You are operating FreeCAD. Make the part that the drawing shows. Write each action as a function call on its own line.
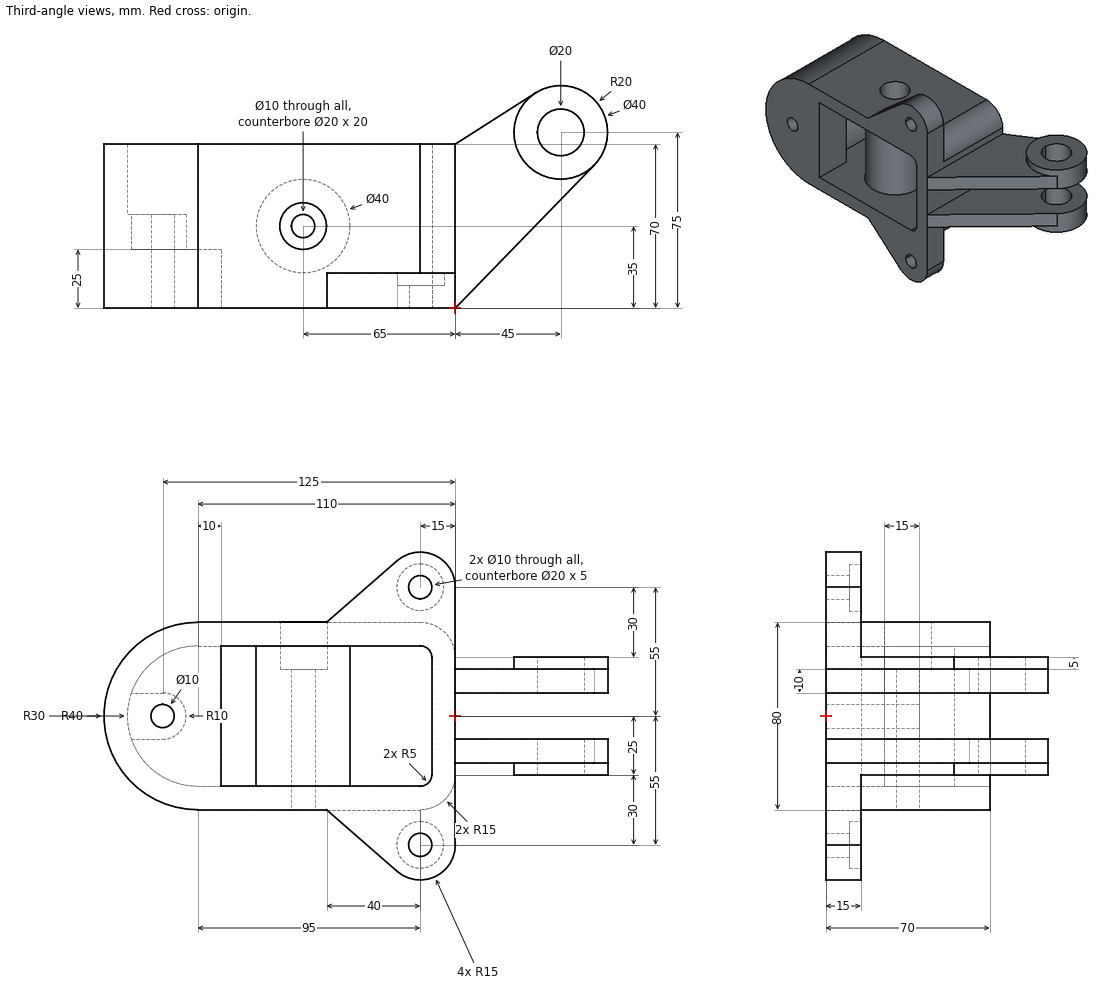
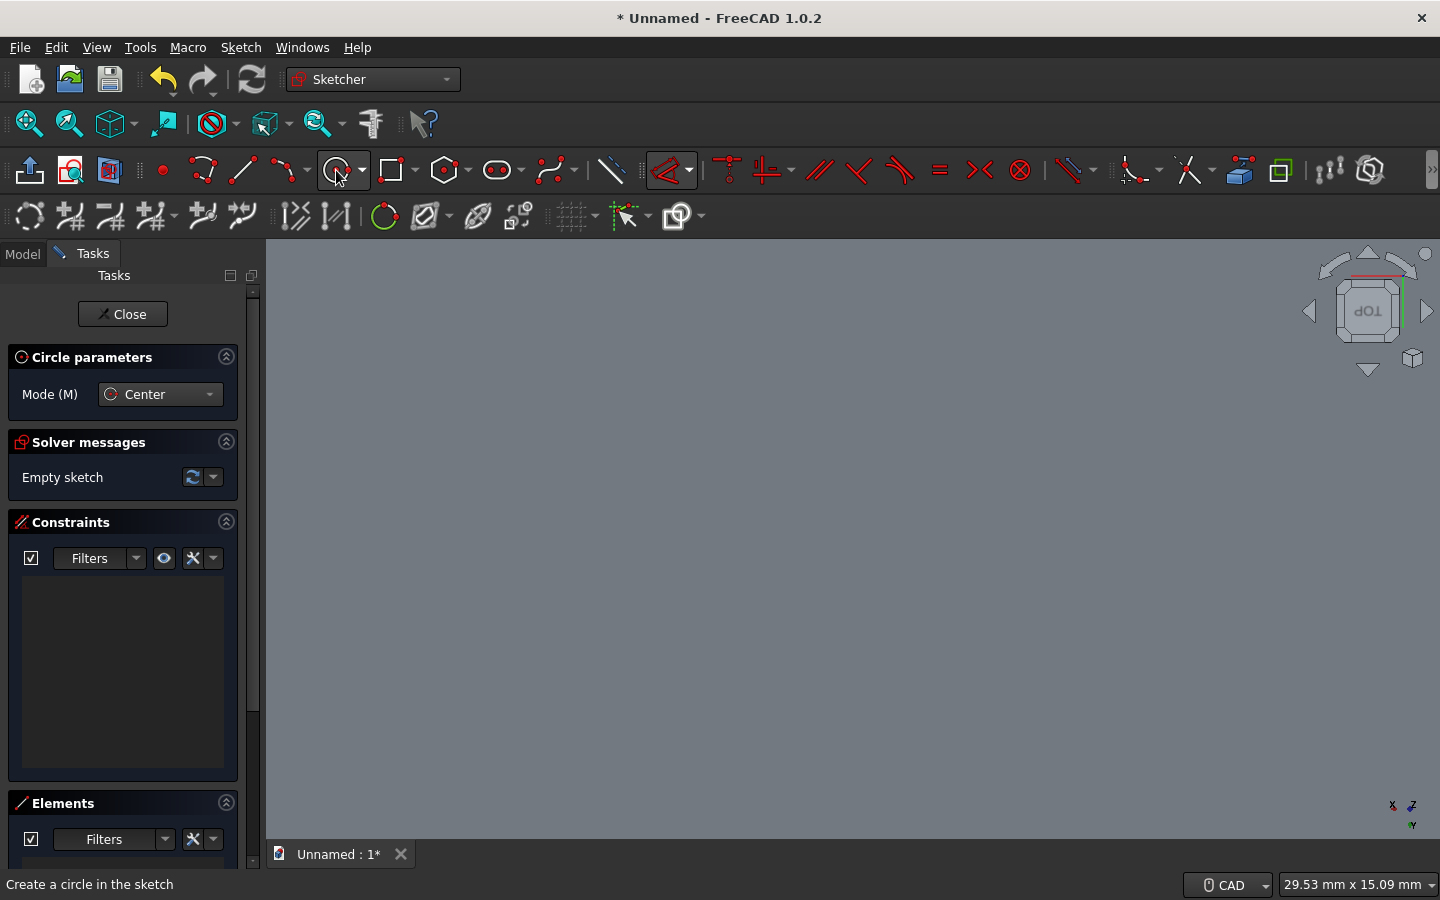
click(773, 535)
move(913, 395)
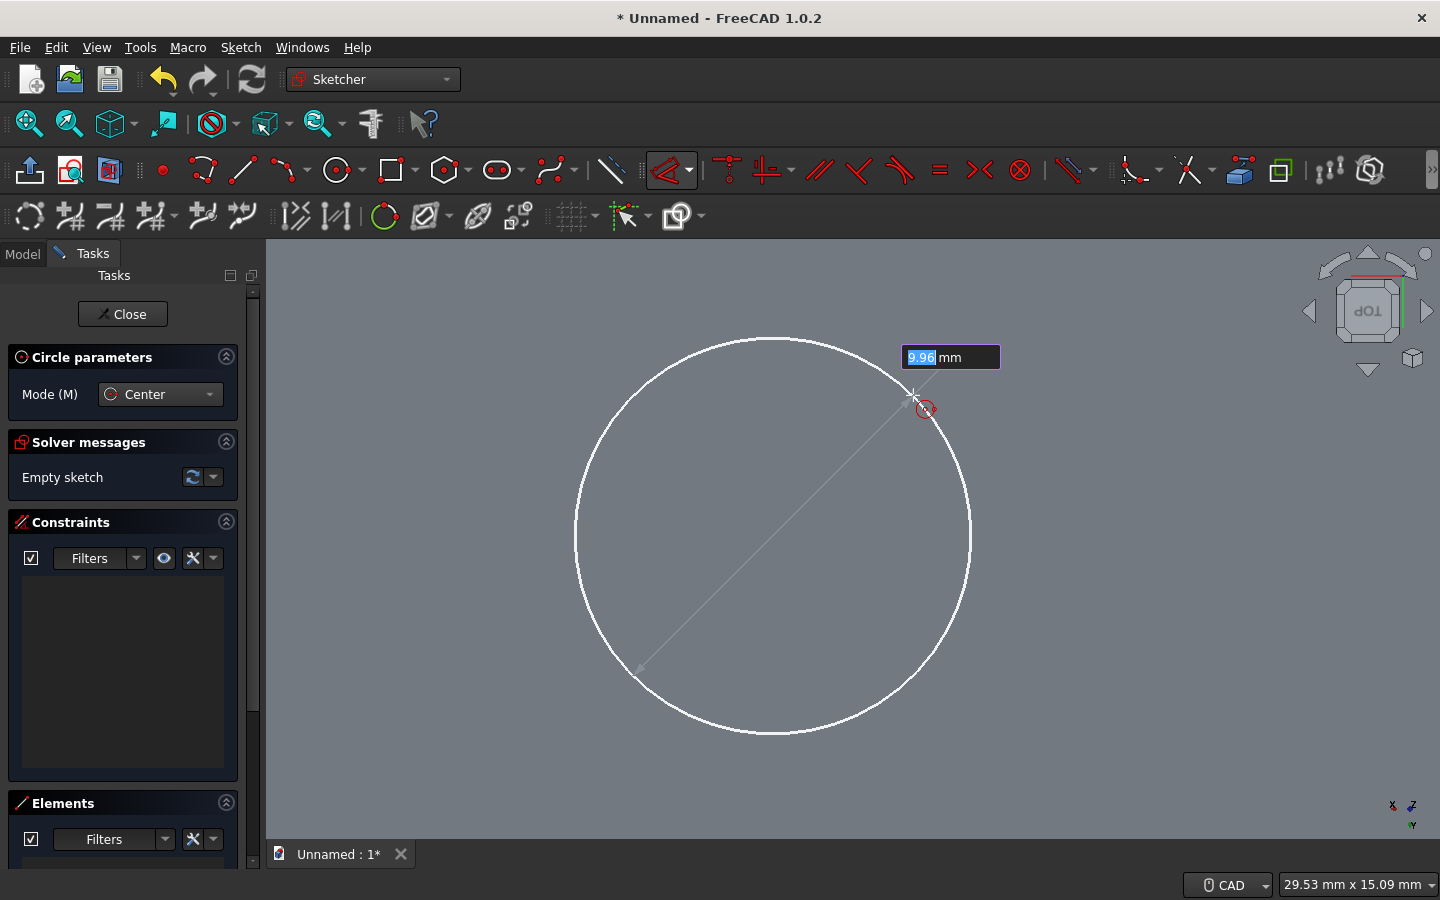
text(10)
key(Return)
key(Escape)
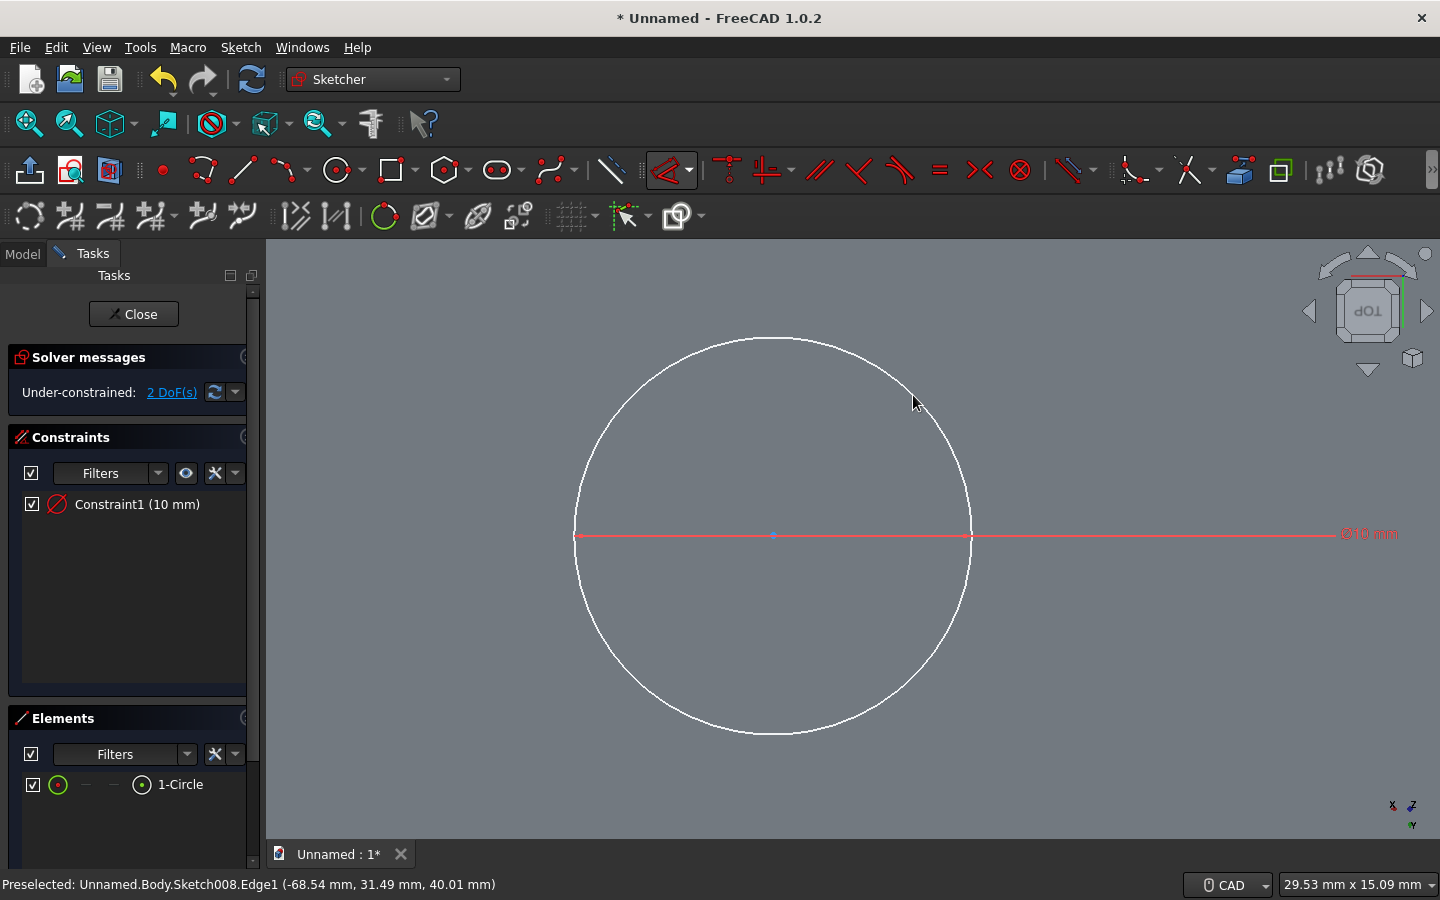
click(773, 536)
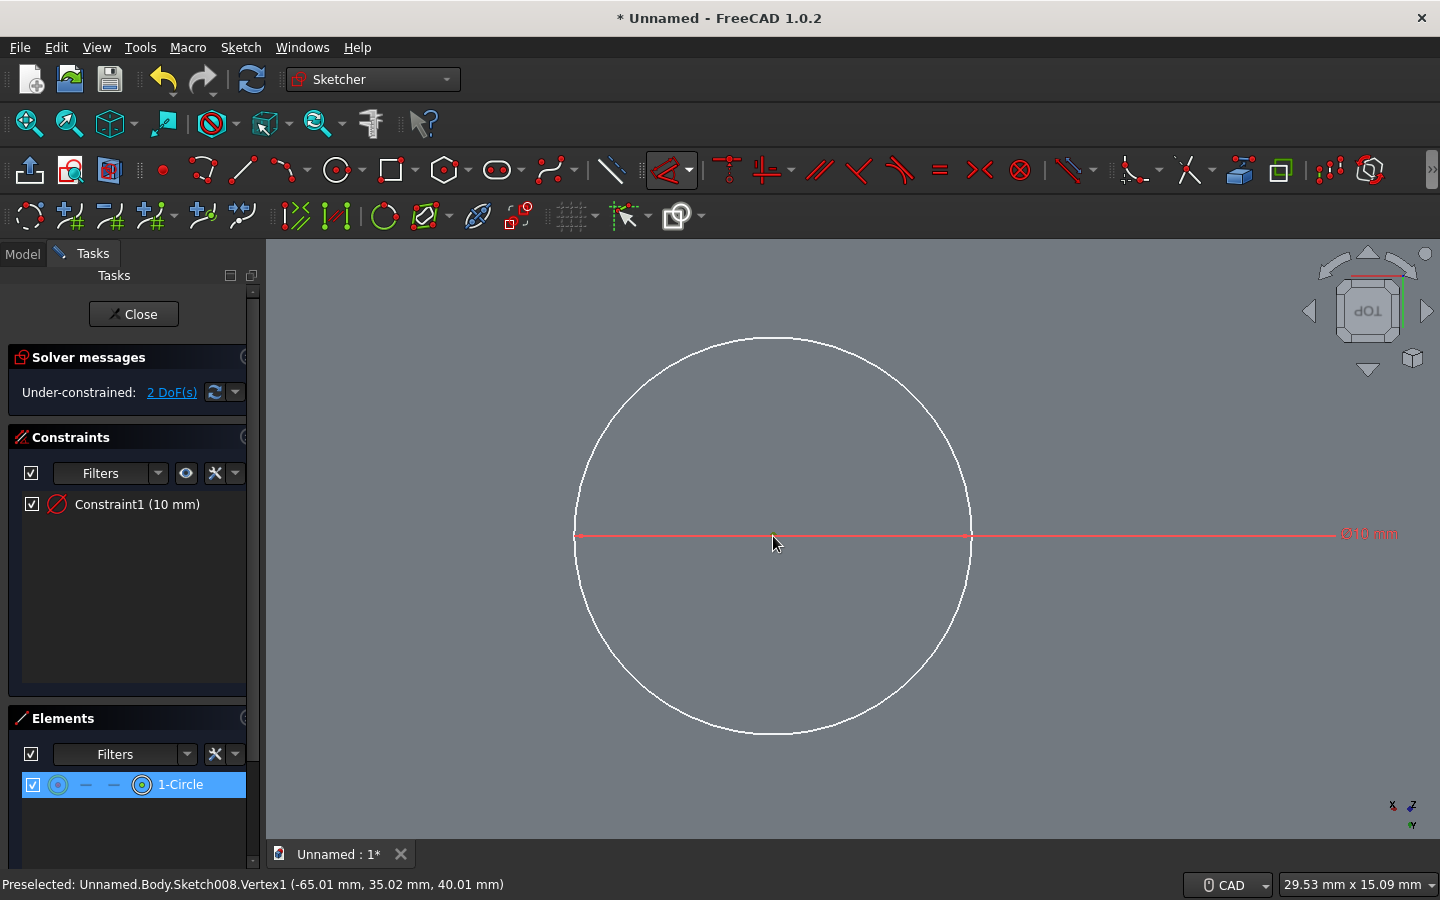
key(l)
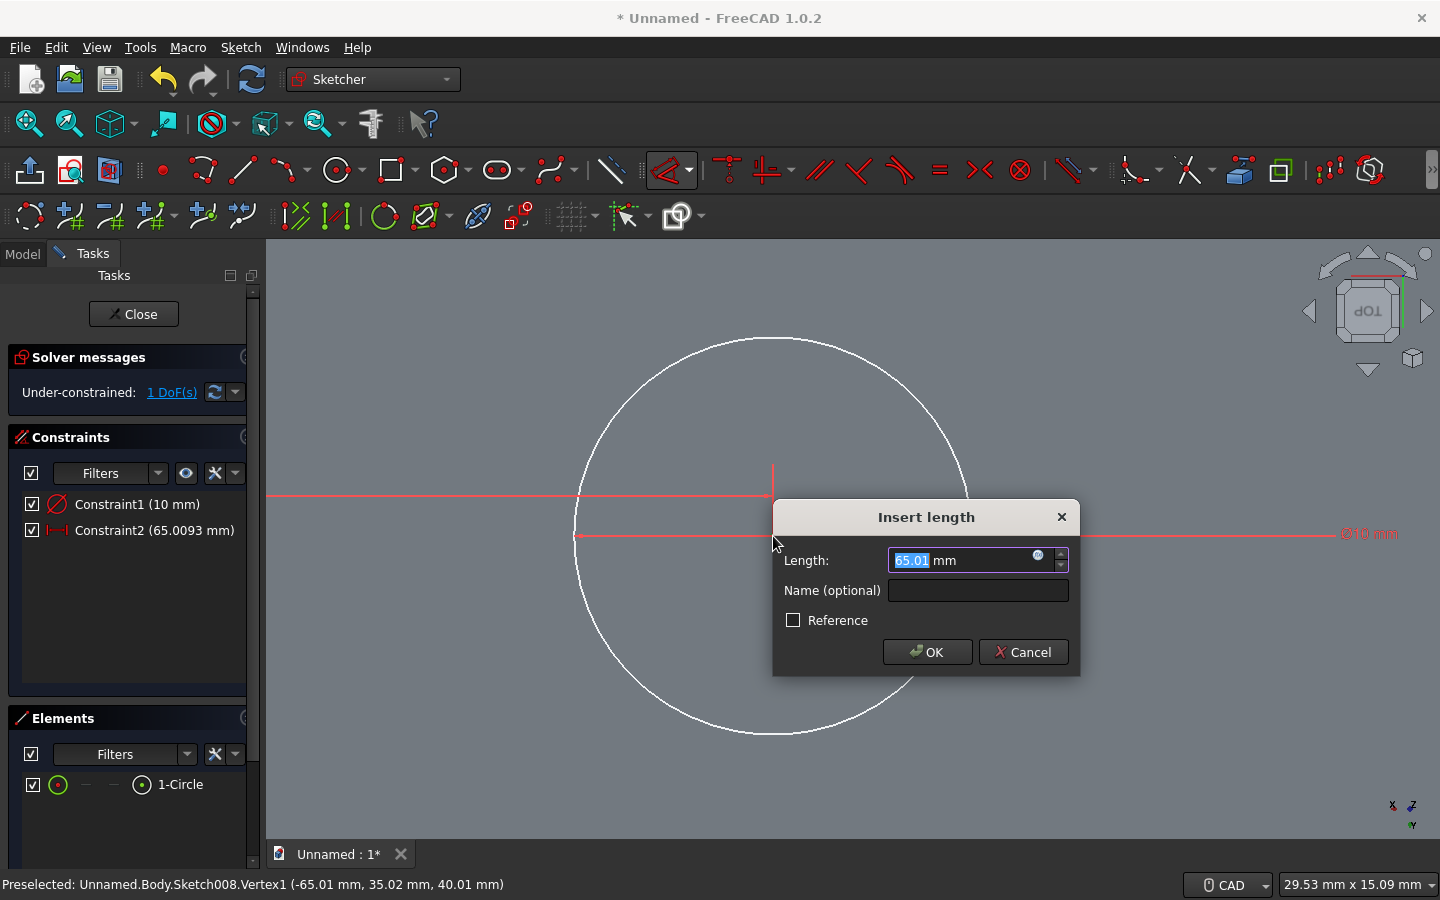
text(65)
key(Return)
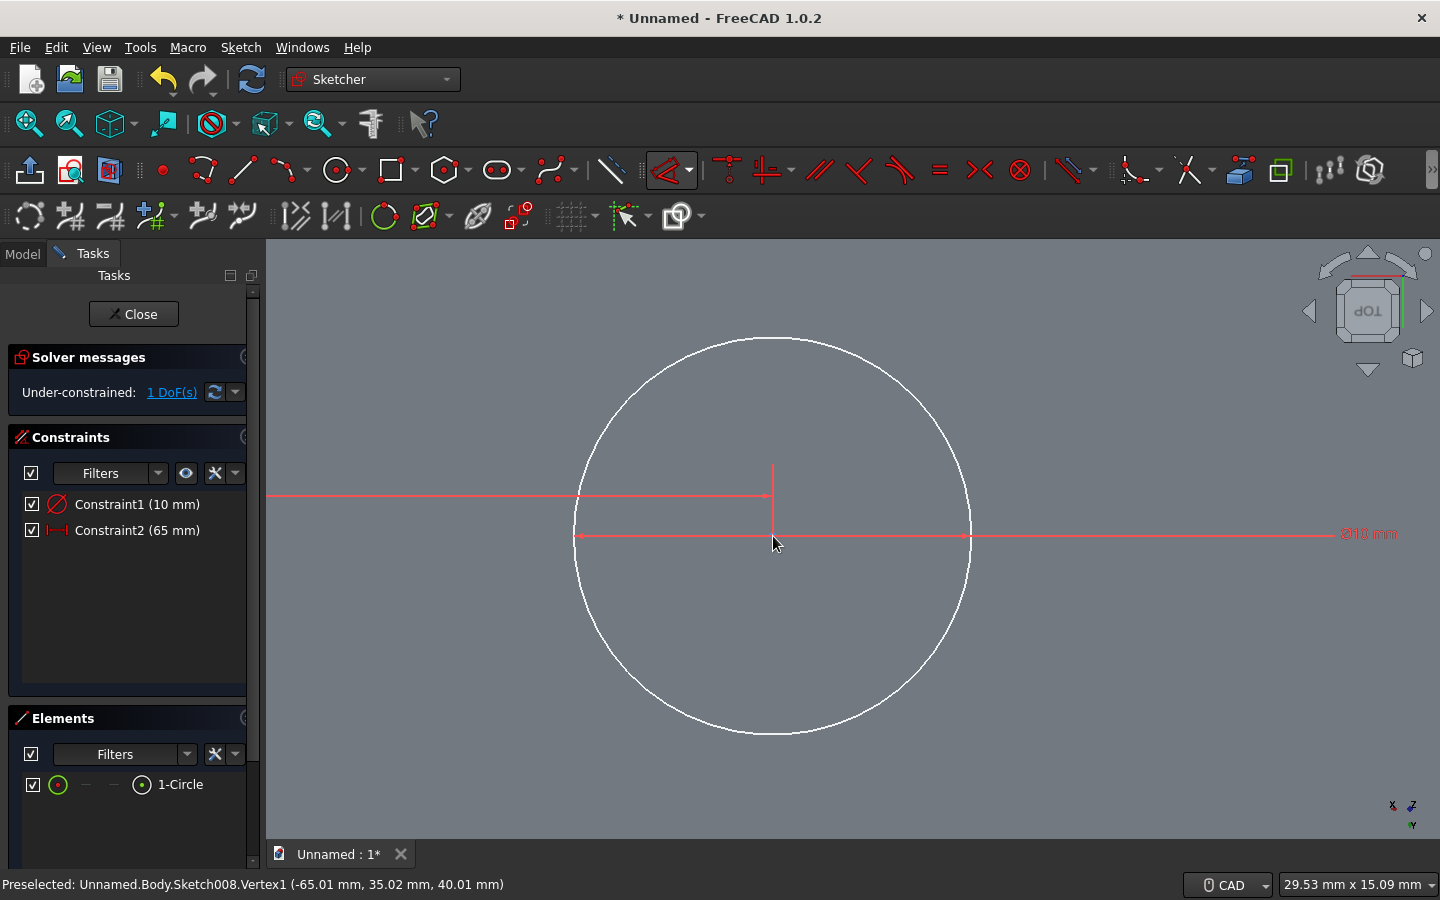
click(773, 536)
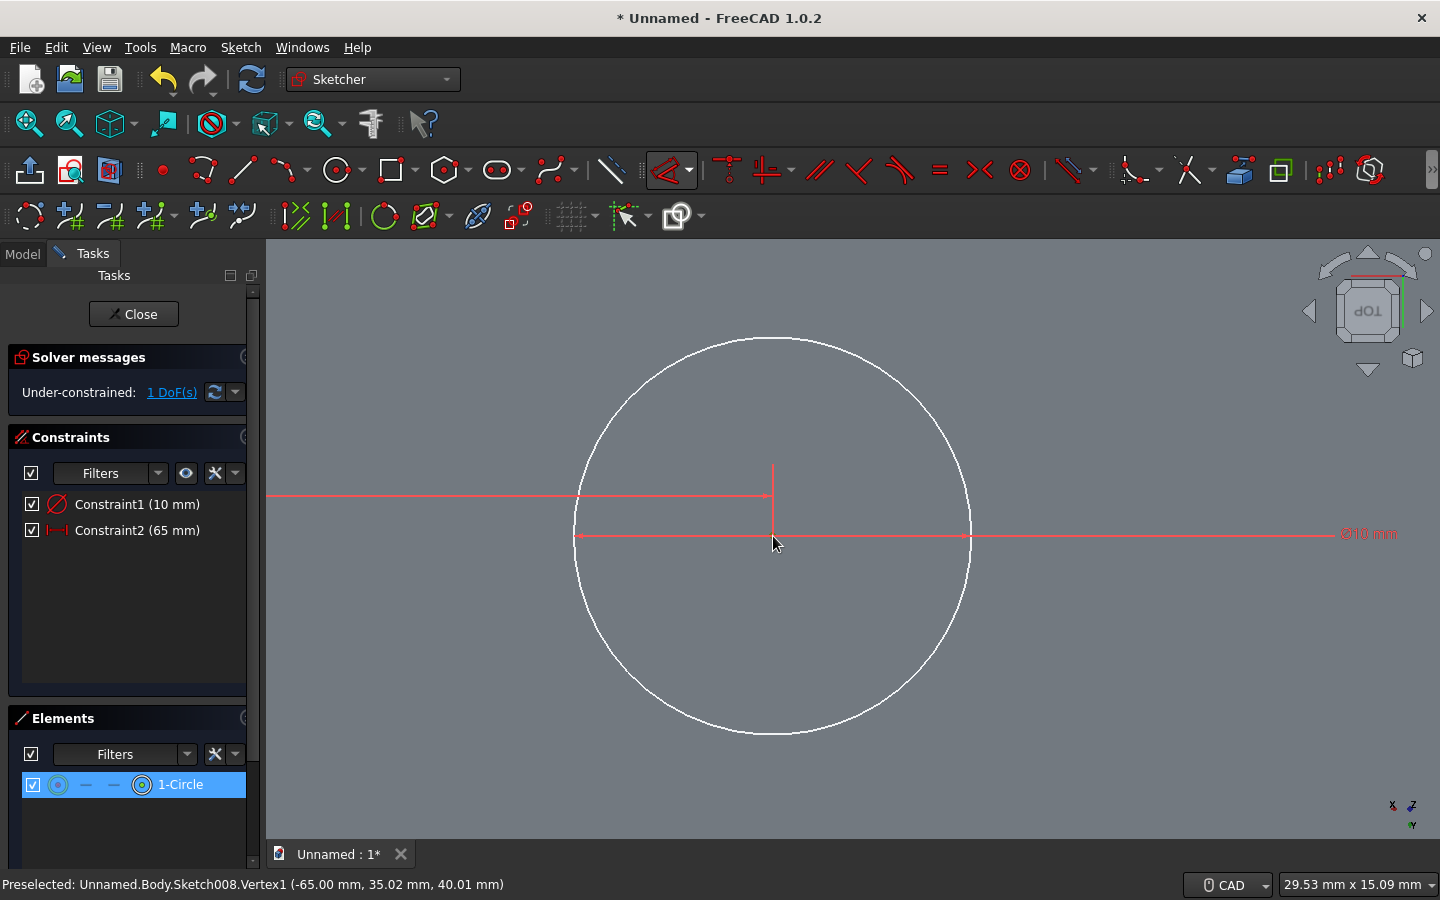
key(i)